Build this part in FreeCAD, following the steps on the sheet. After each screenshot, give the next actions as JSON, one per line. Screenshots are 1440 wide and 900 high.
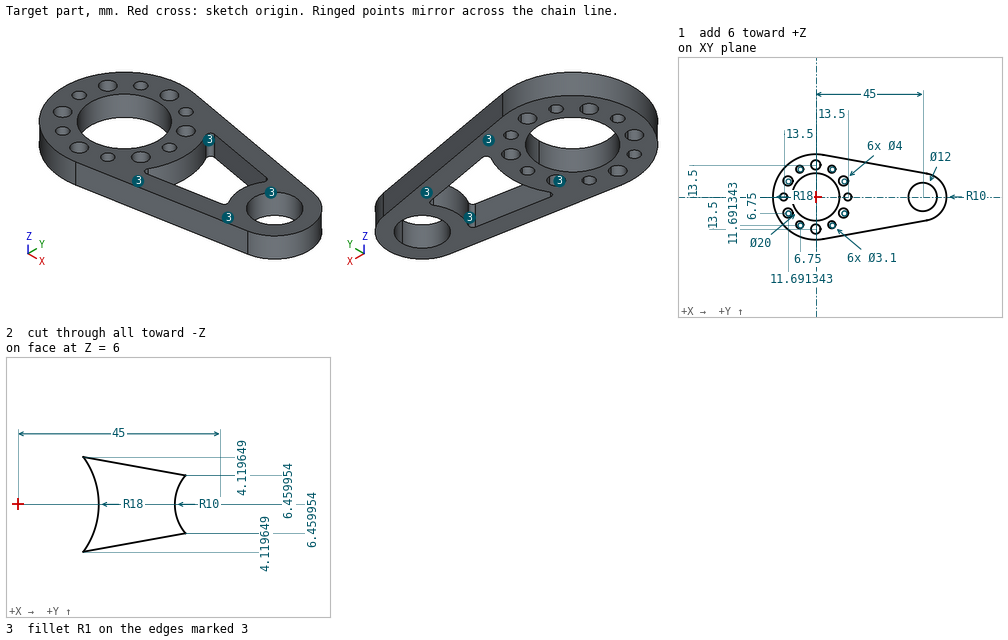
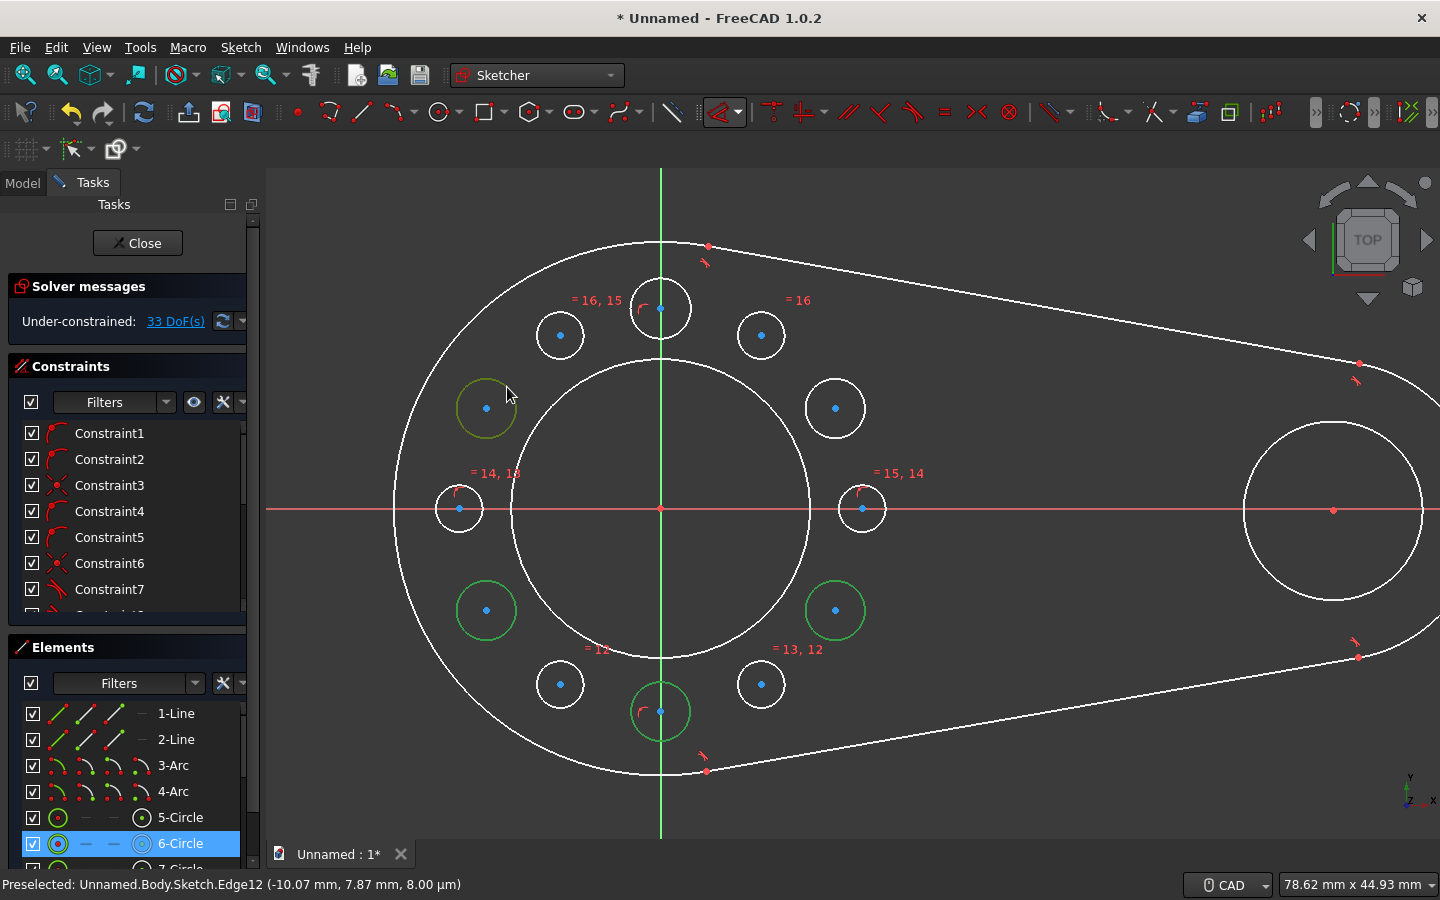
{"action": "left_click", "coordinate": [856, 387]}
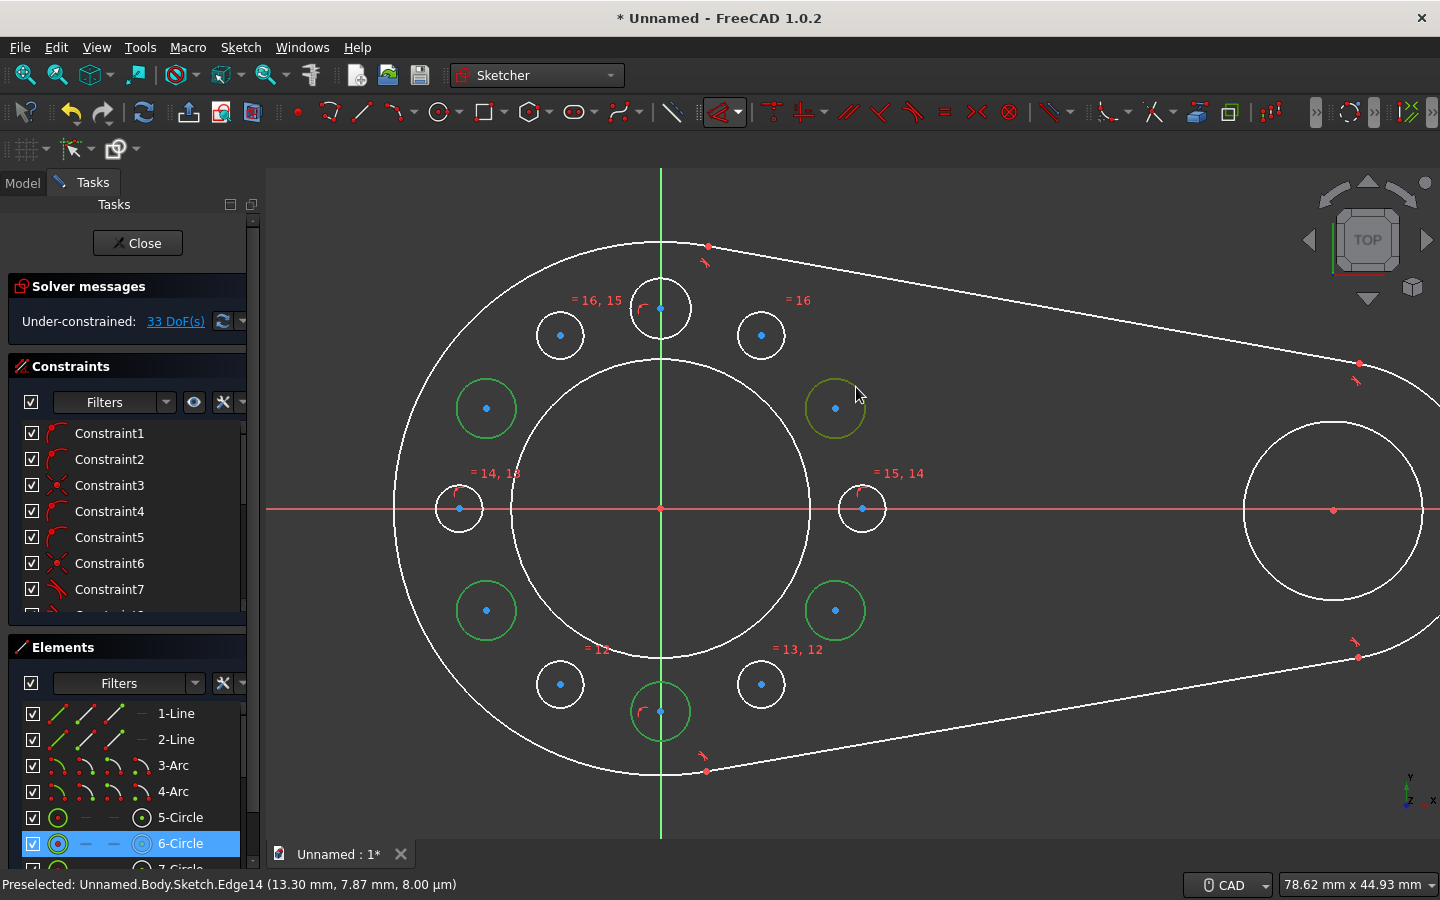
{"action": "left_click", "coordinate": [682, 287]}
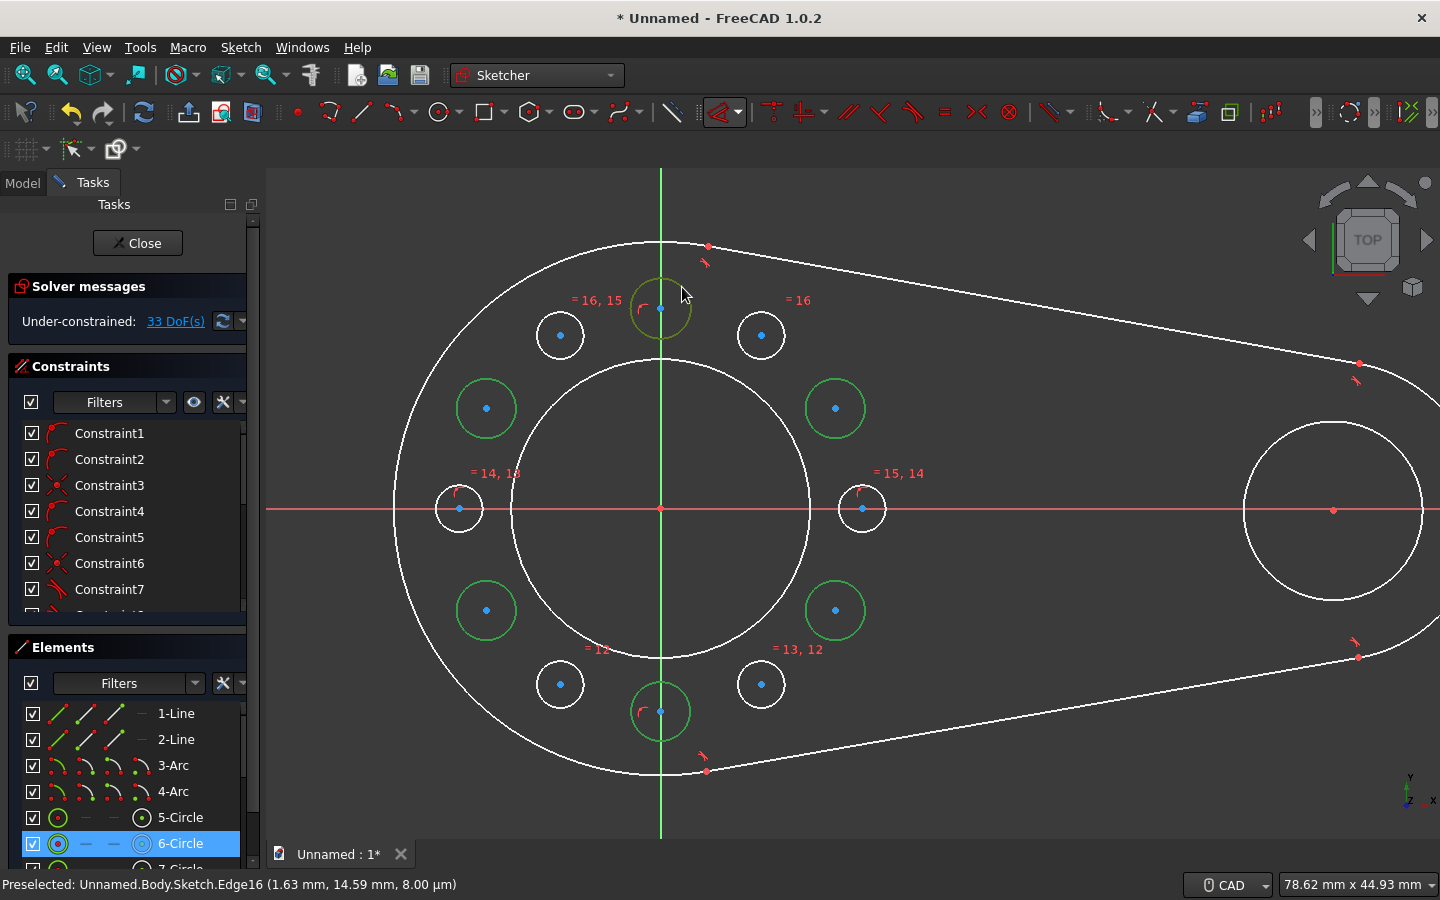
{"action": "left_click", "coordinate": [946, 112]}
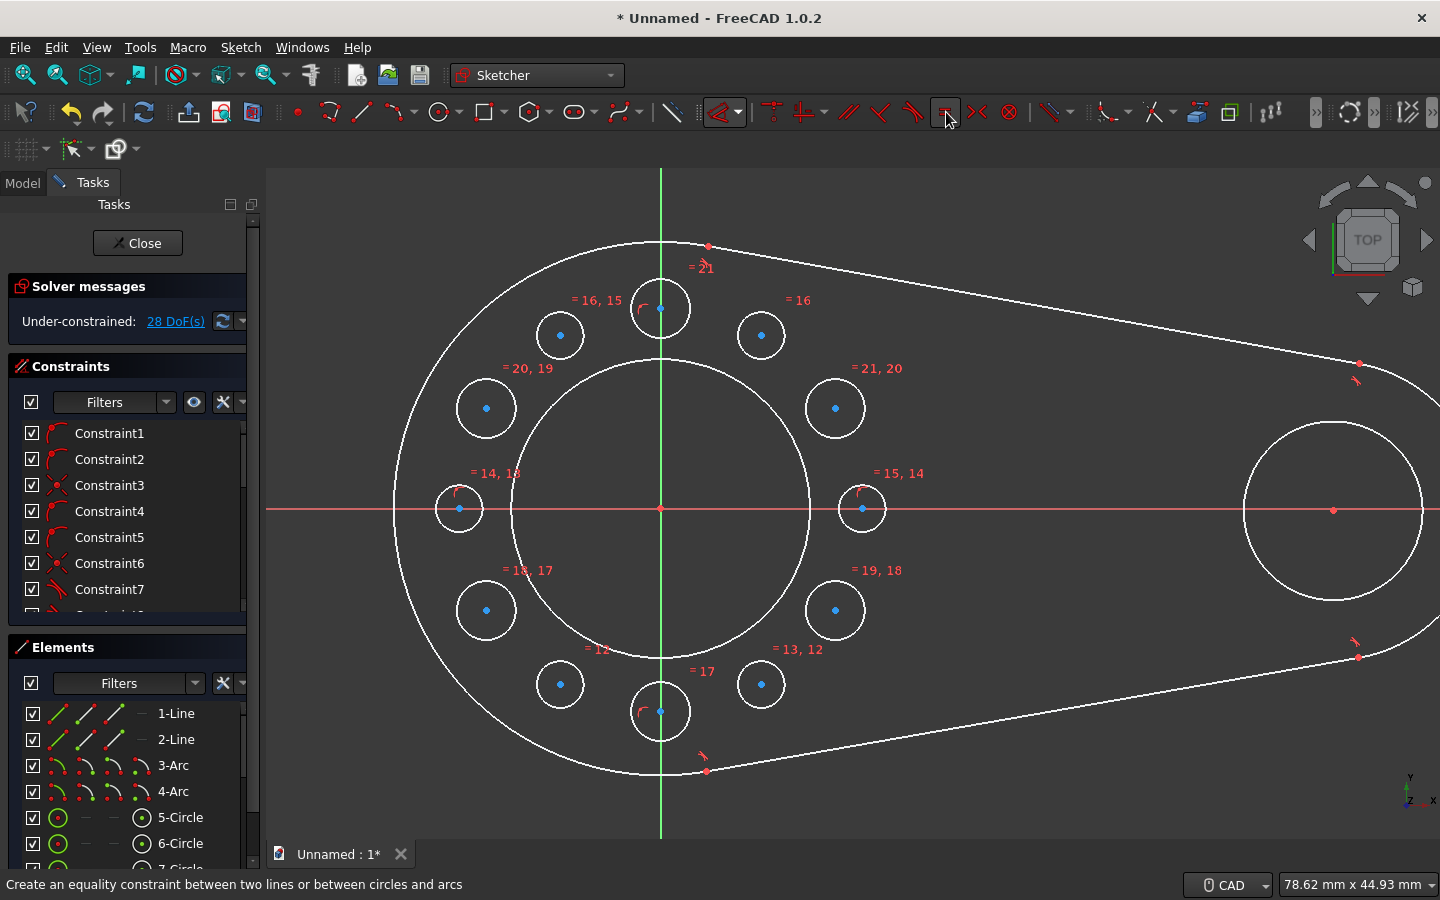
{"action": "scroll", "coordinate": [475, 493], "scroll_direction": "down", "scroll_amount": 2}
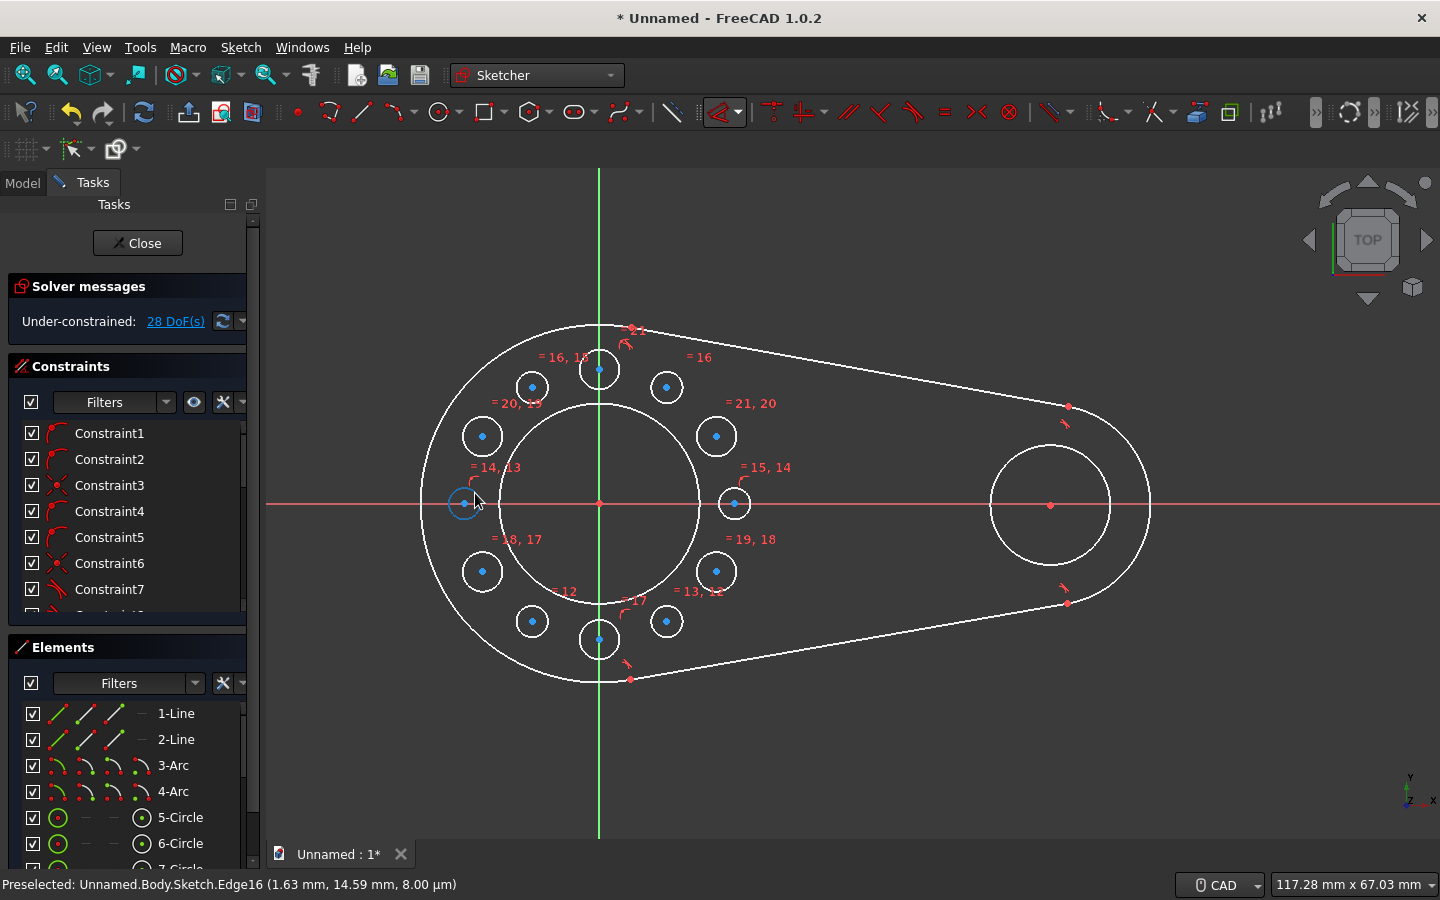
{"action": "left_click", "coordinate": [1050, 505]}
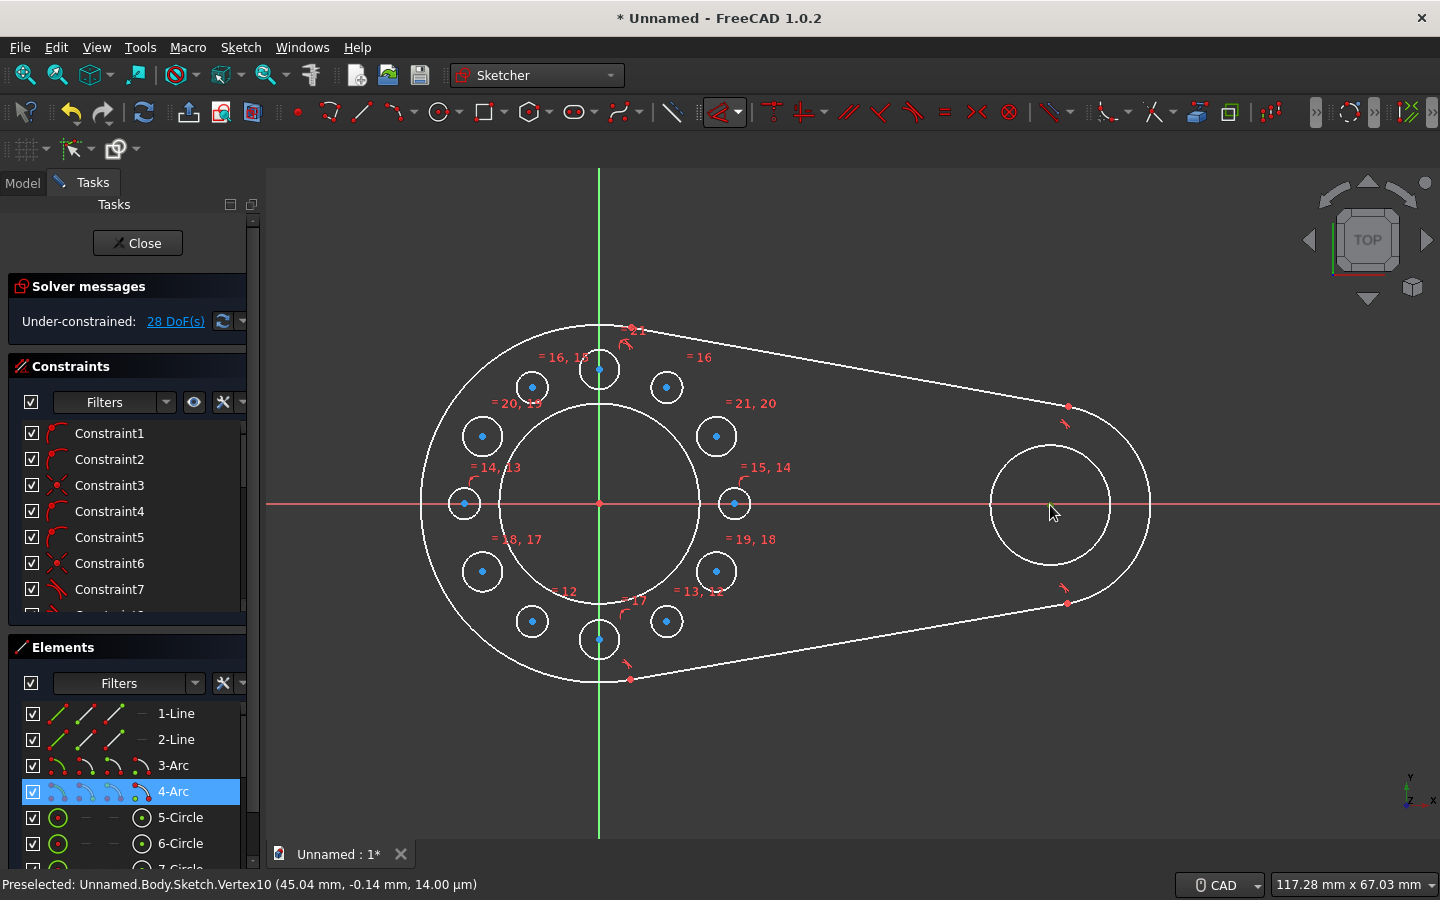
{"action": "left_click", "coordinate": [364, 504]}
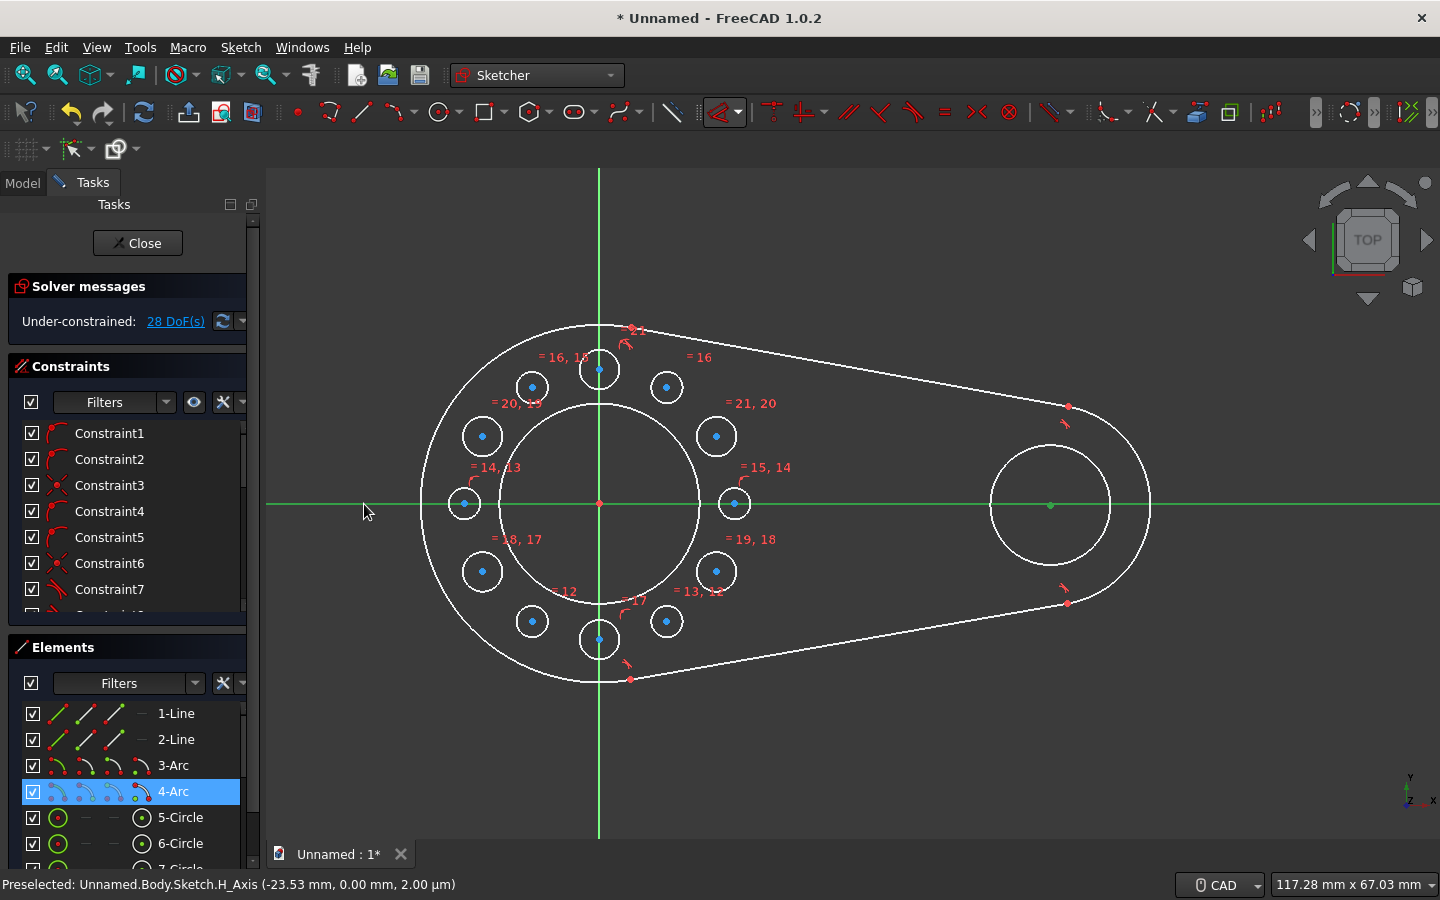
{"action": "key", "text": "c"}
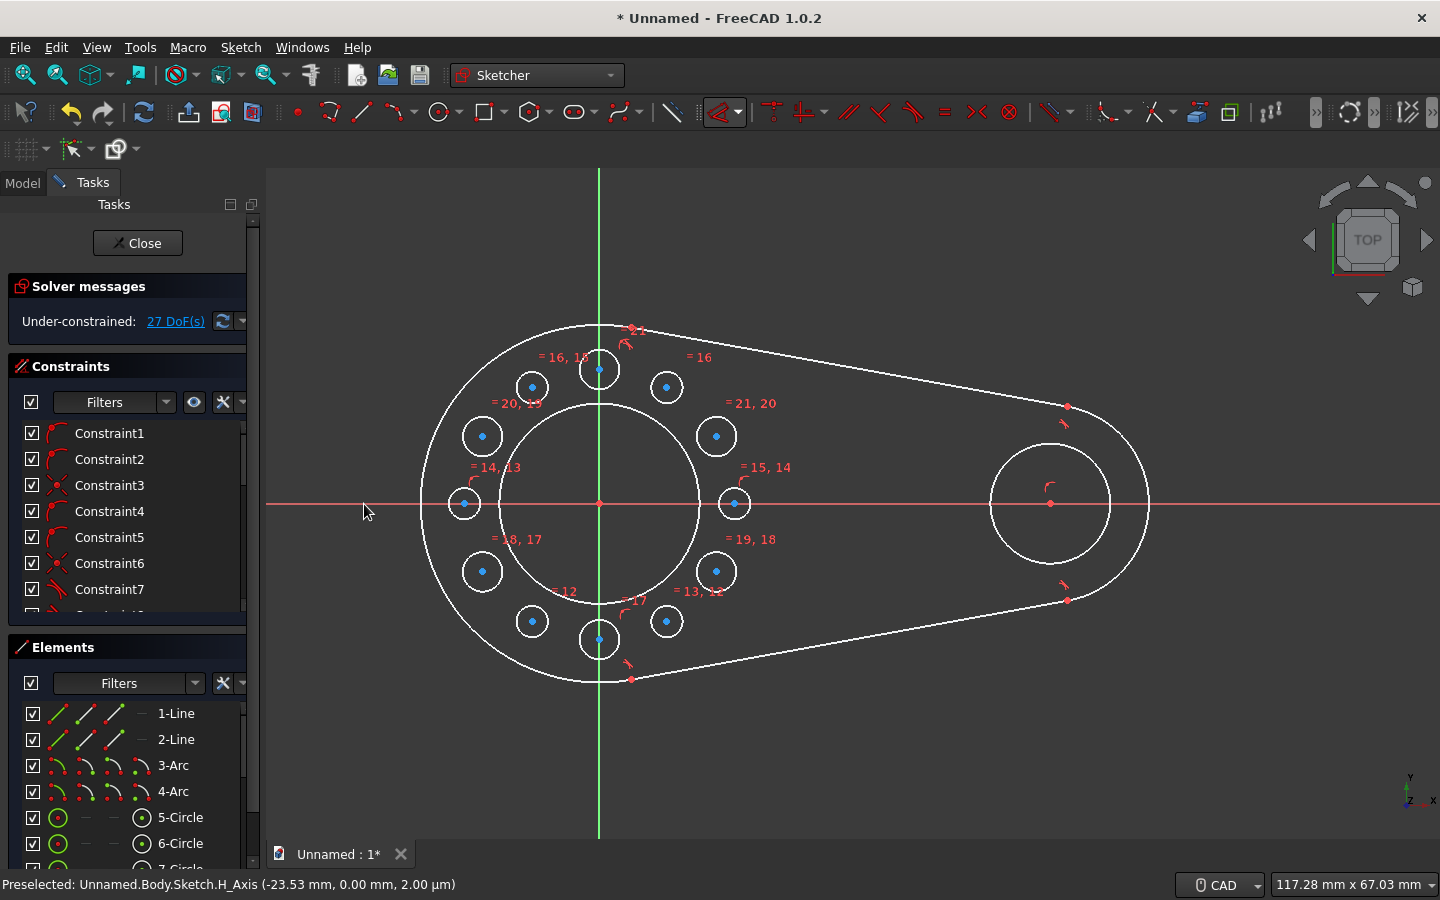
{"action": "left_click", "coordinate": [532, 622]}